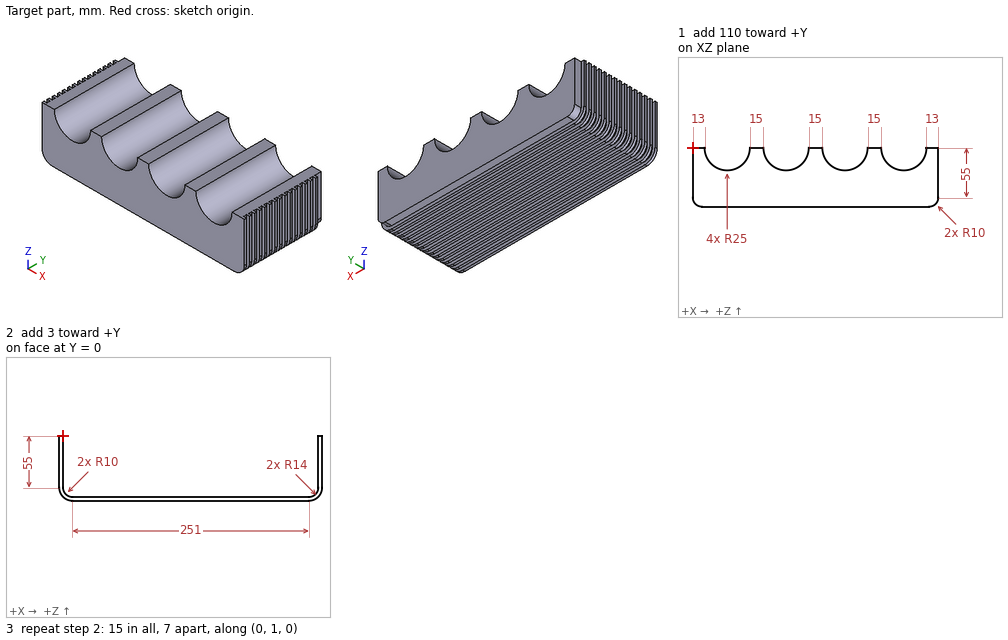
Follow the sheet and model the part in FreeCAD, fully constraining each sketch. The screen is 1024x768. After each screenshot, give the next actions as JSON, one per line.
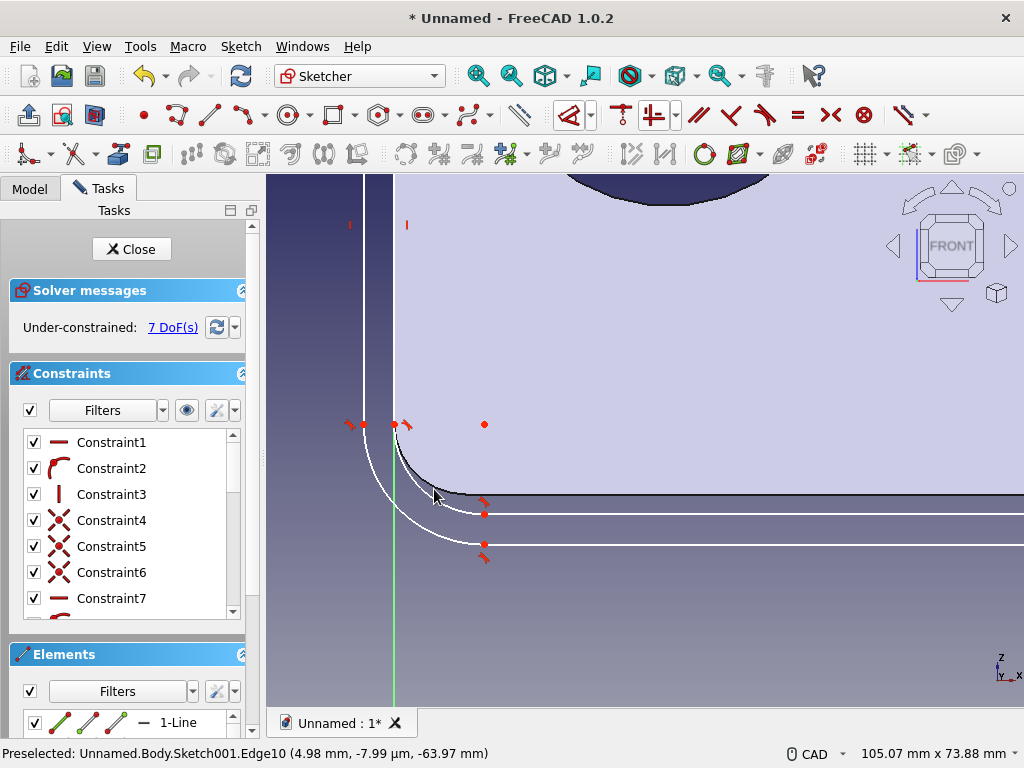
{"action": "scroll", "coordinate": [375, 482], "scroll_direction": "down", "scroll_amount": 8}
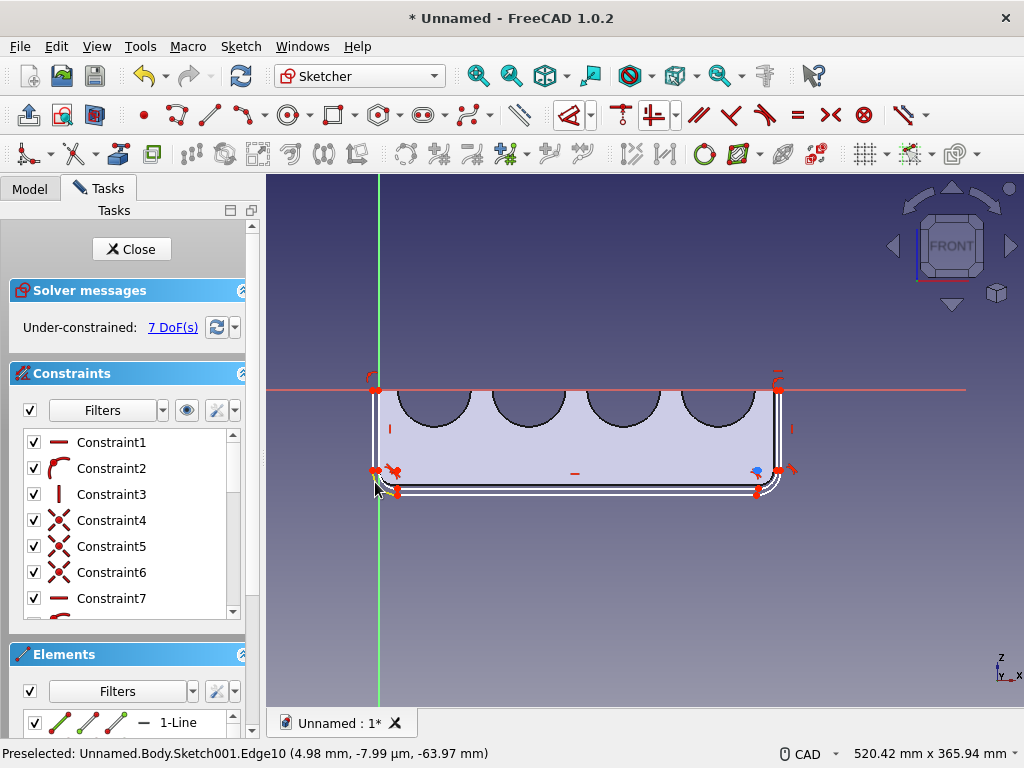
{"action": "scroll", "coordinate": [767, 487], "scroll_direction": "up", "scroll_amount": 6}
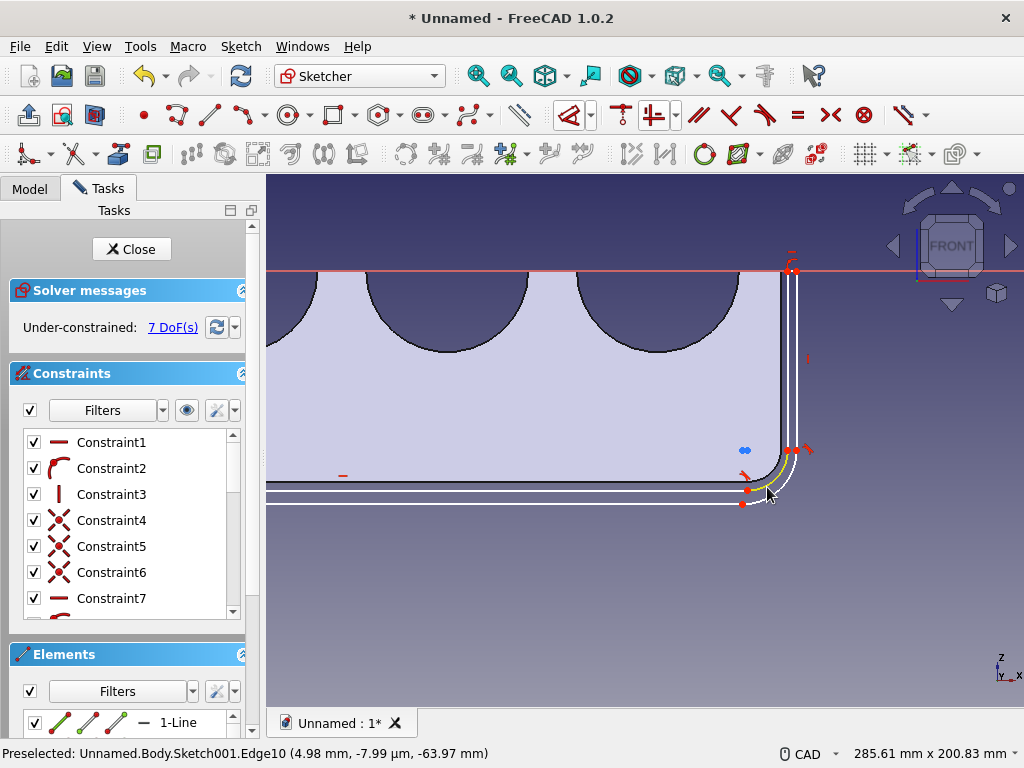
{"action": "left_click", "coordinate": [765, 486]}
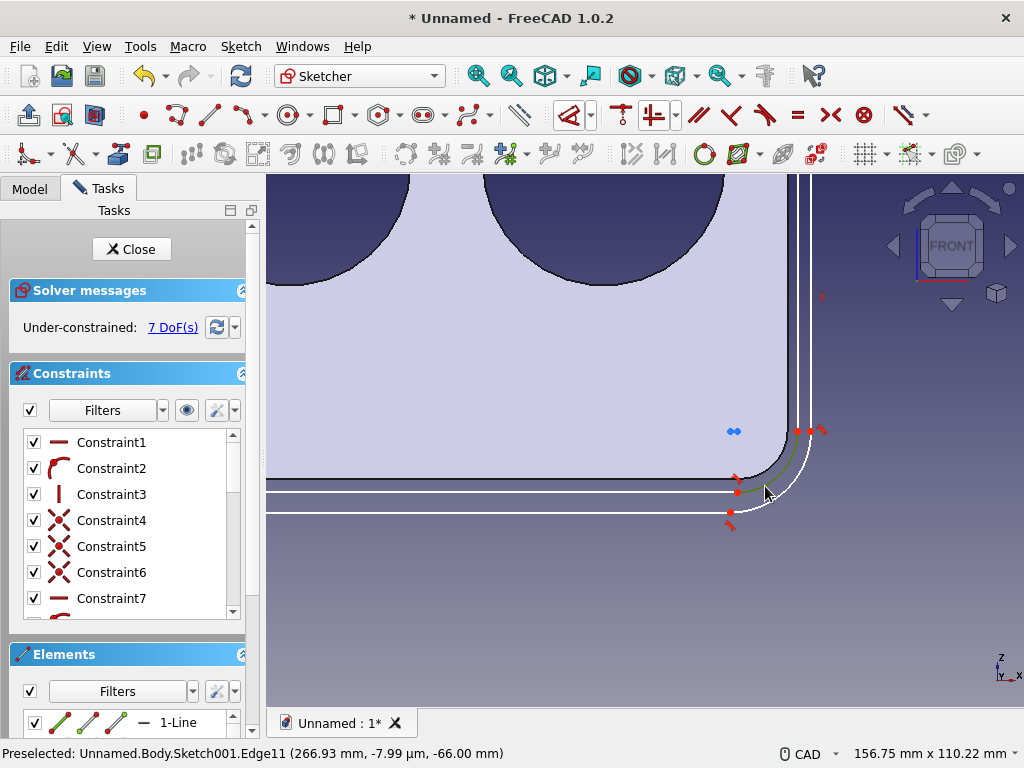
{"action": "left_click", "coordinate": [767, 504]}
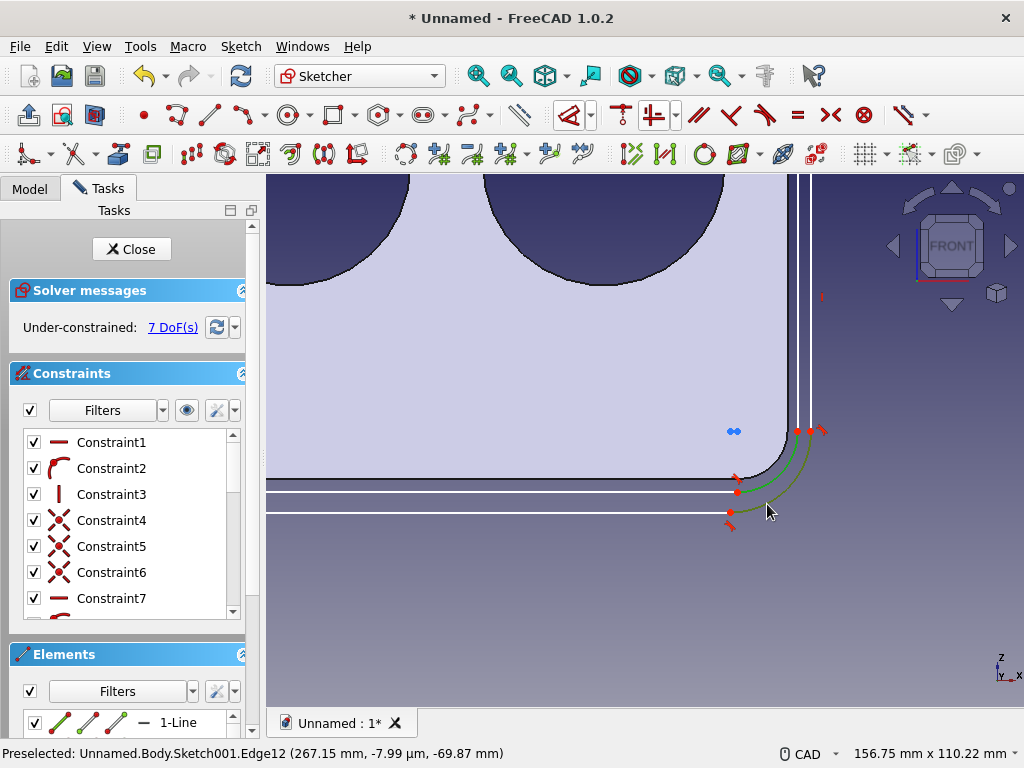
{"action": "left_click", "coordinate": [621, 116]}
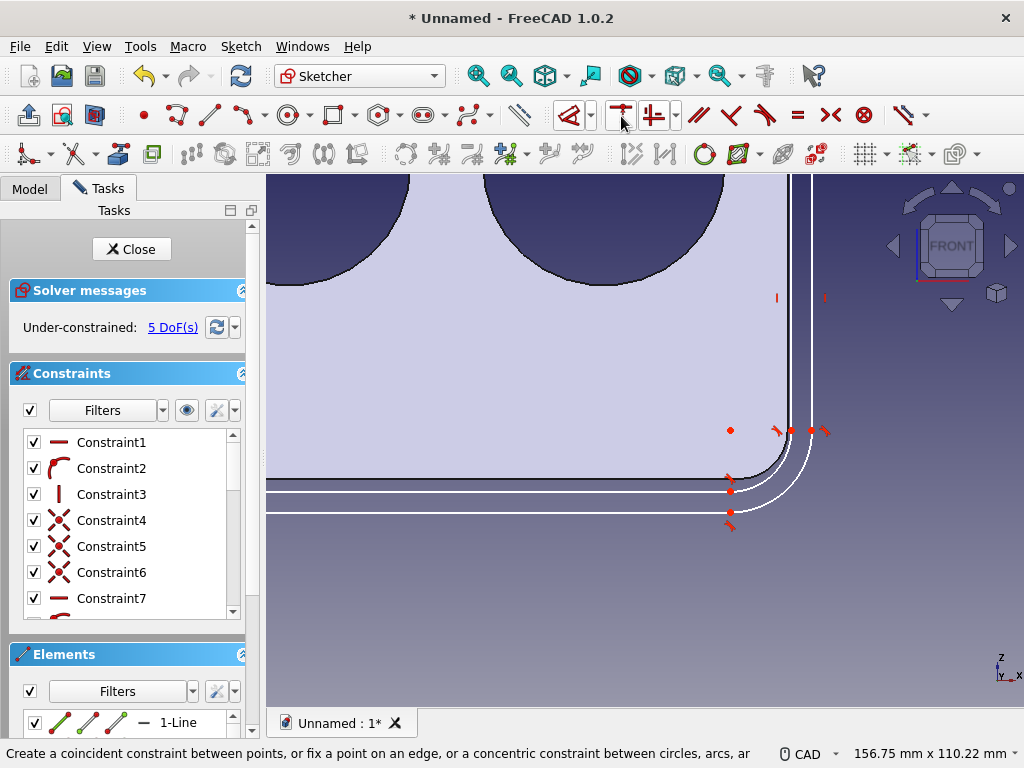
{"action": "scroll", "coordinate": [768, 487], "scroll_direction": "down", "scroll_amount": 6}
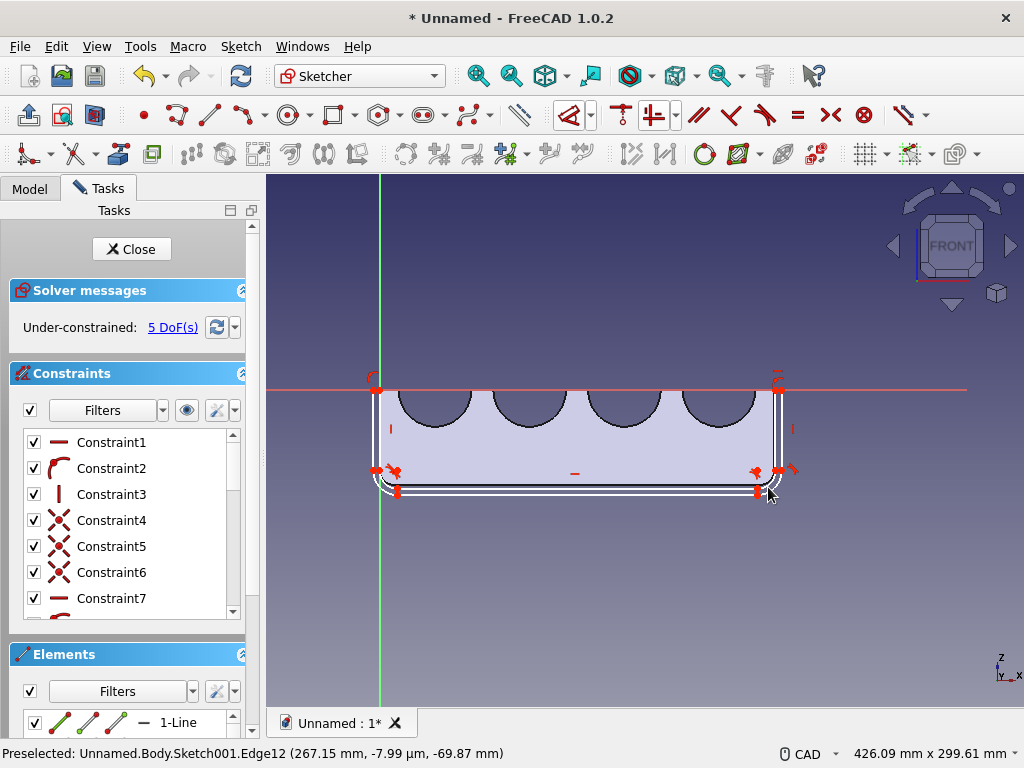
{"action": "scroll", "coordinate": [390, 487], "scroll_direction": "up", "scroll_amount": 4}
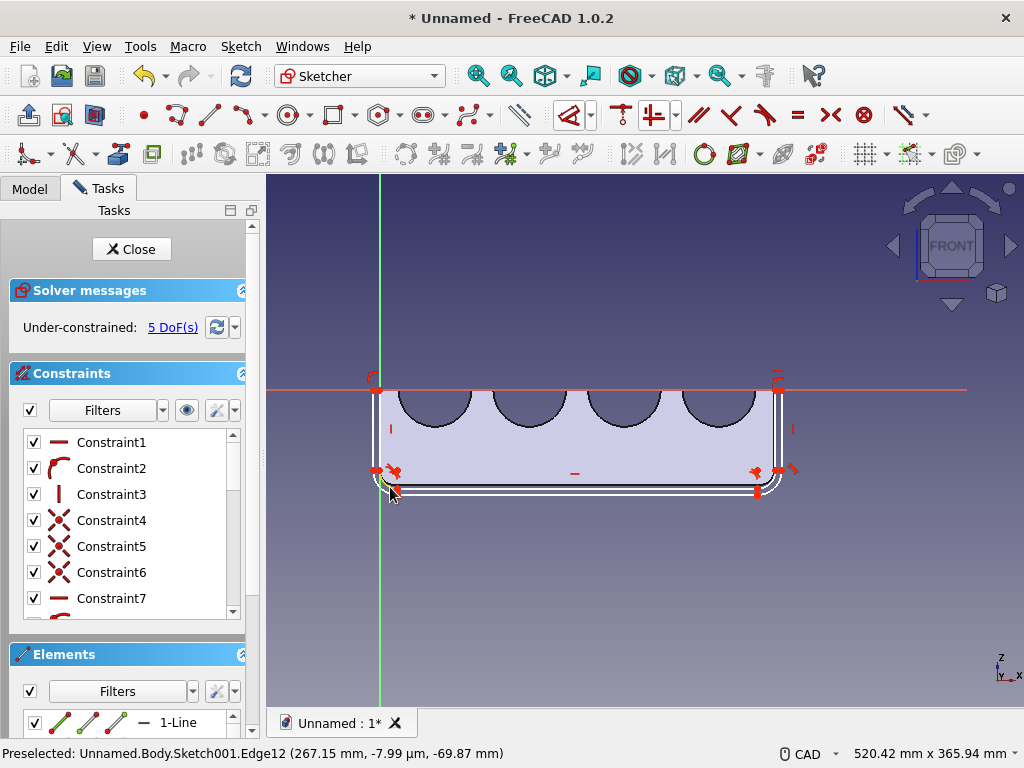
{"action": "left_click", "coordinate": [389, 486]}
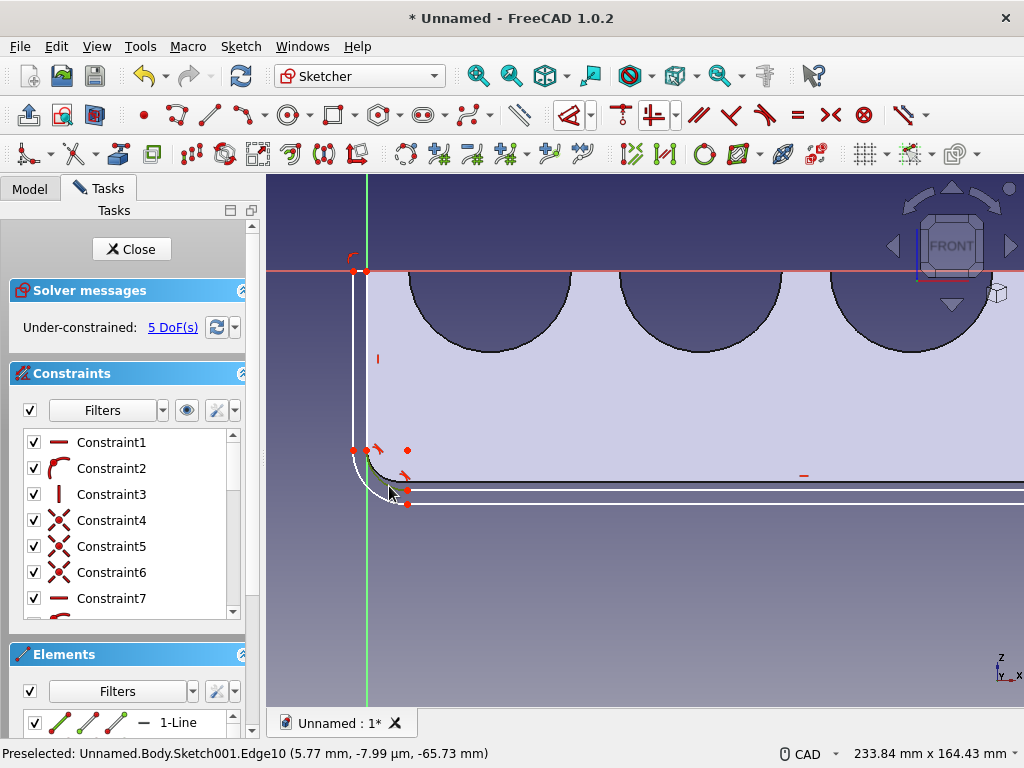
{"action": "scroll", "coordinate": [389, 487], "scroll_direction": "down", "scroll_amount": 4}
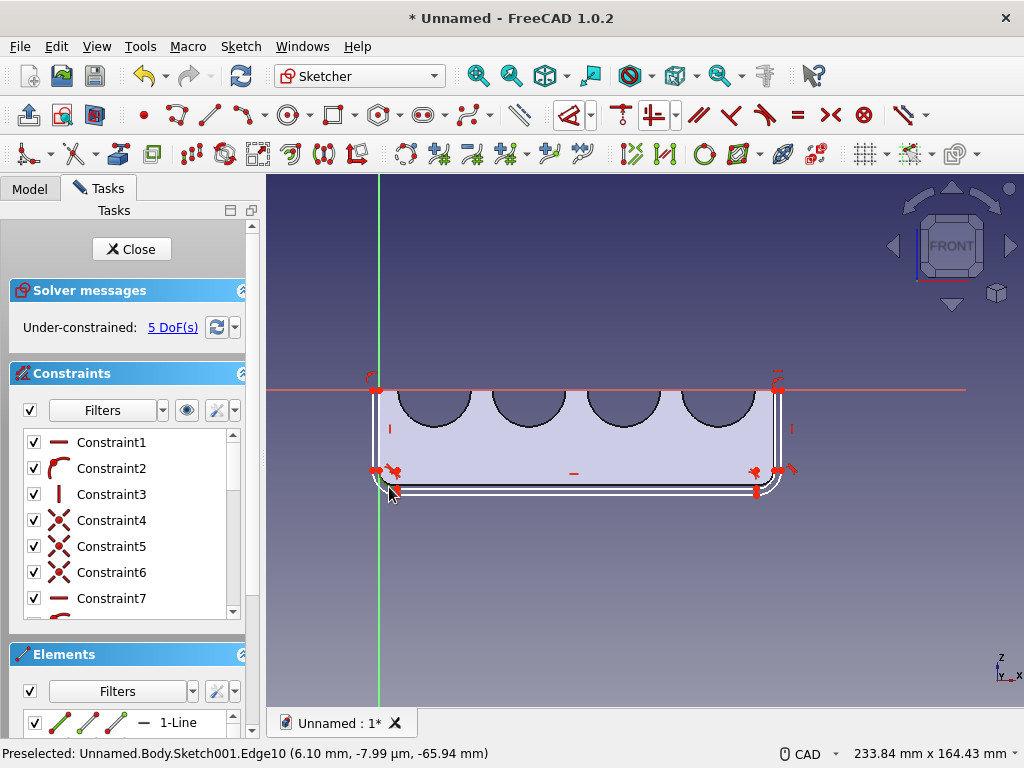
{"action": "scroll", "coordinate": [765, 487], "scroll_direction": "up", "scroll_amount": 4}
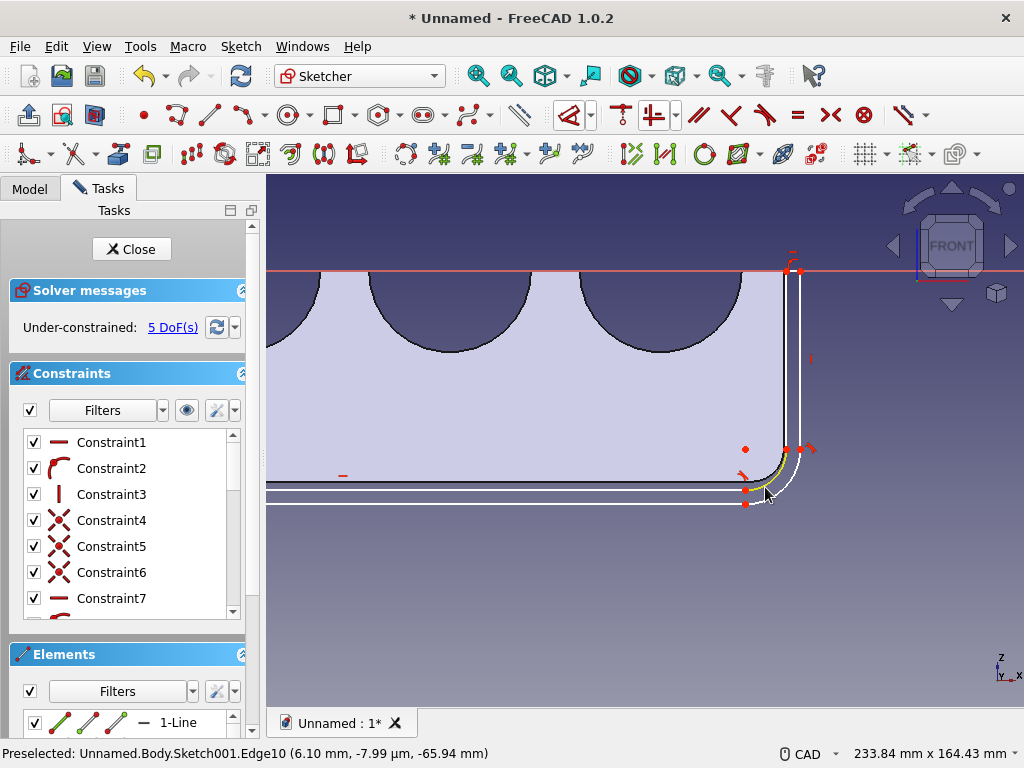
{"action": "left_click", "coordinate": [764, 486]}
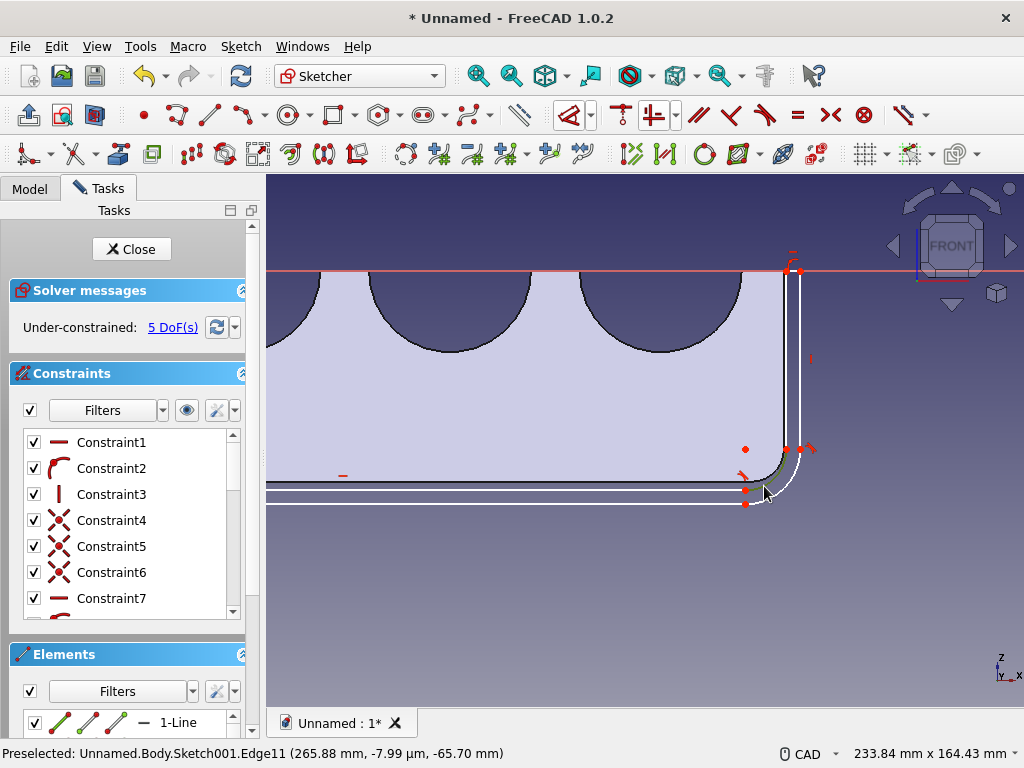
{"action": "key", "text": "e"}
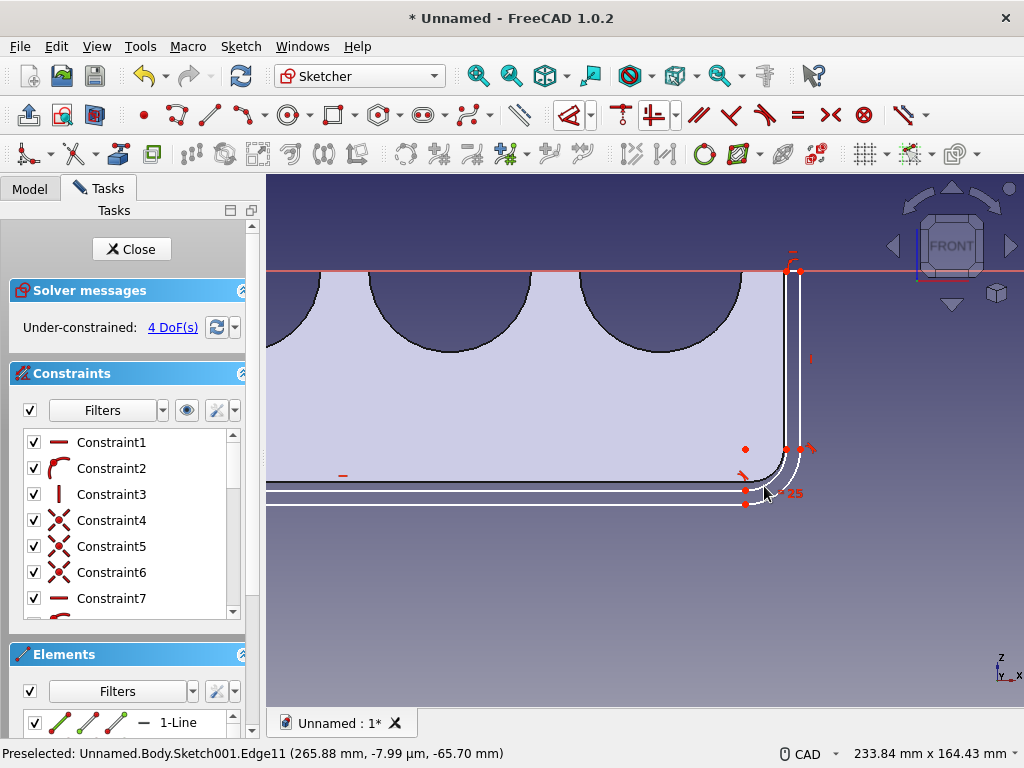
{"action": "scroll", "coordinate": [766, 487], "scroll_direction": "down", "scroll_amount": 4}